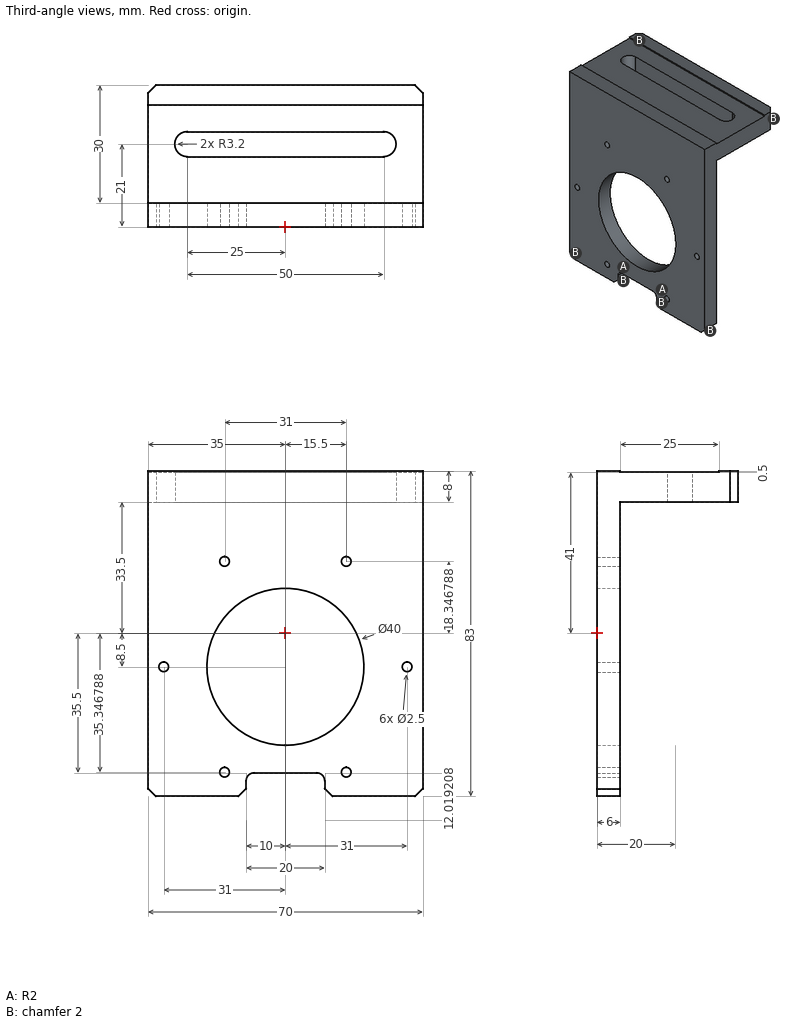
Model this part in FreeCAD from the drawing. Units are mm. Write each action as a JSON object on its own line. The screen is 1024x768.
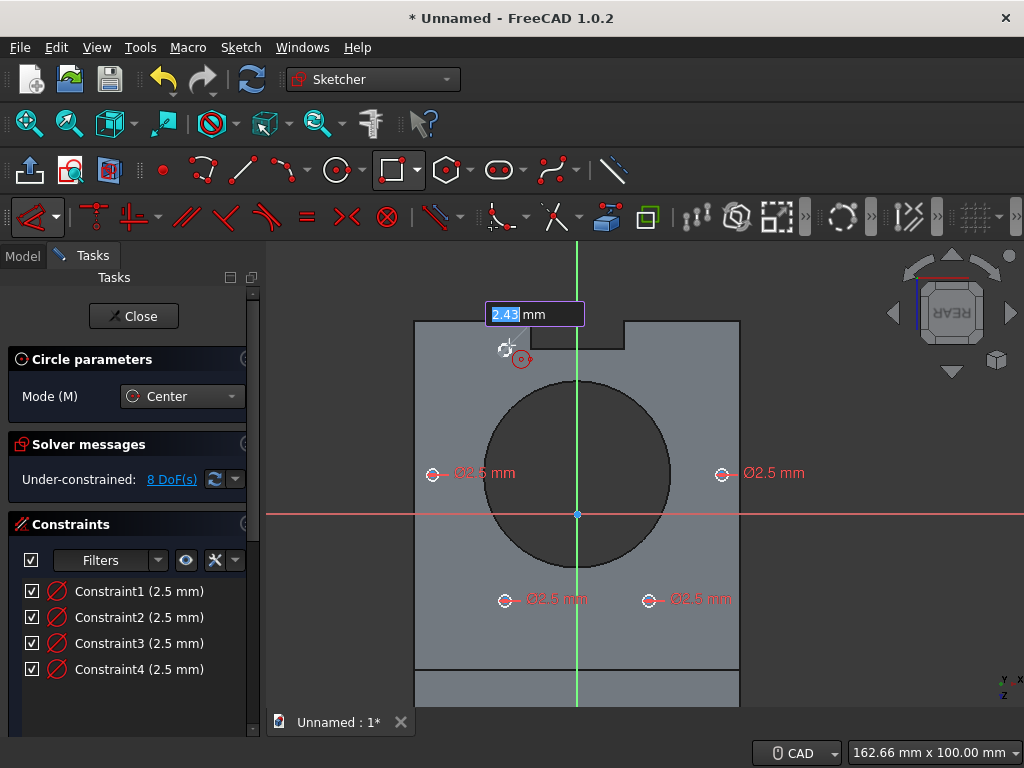
{"action": "type", "text": "2.5"}
{"action": "key", "text": "Return"}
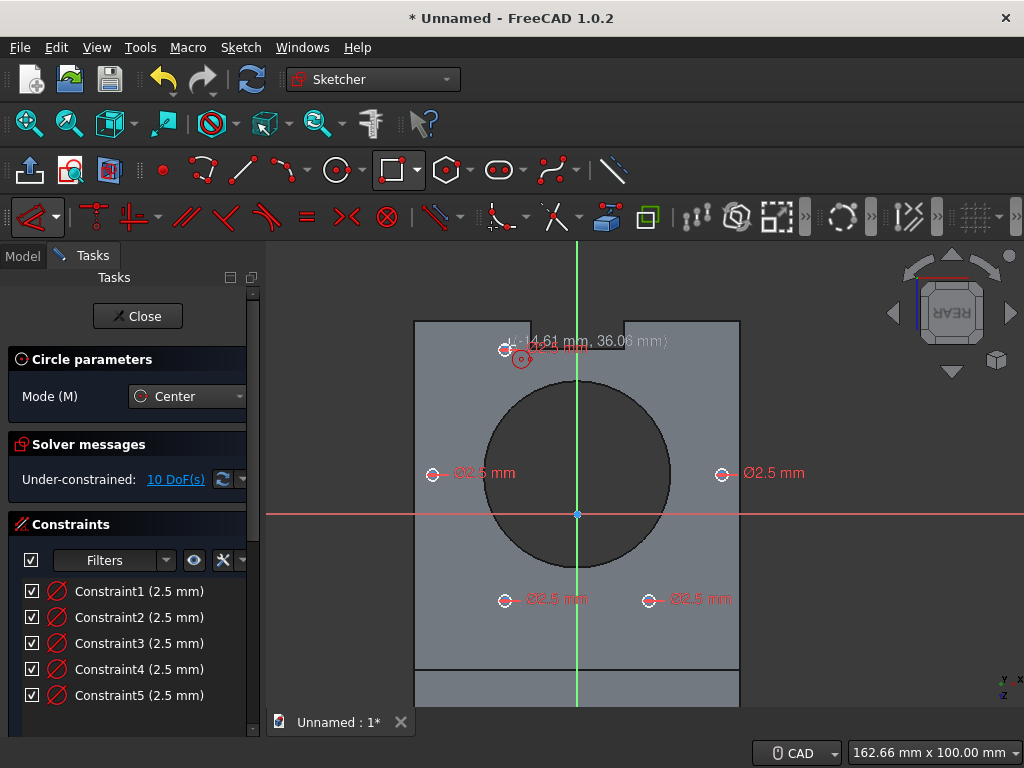
{"action": "scroll", "coordinate": [649, 349], "scroll_direction": "up", "scroll_amount": 7}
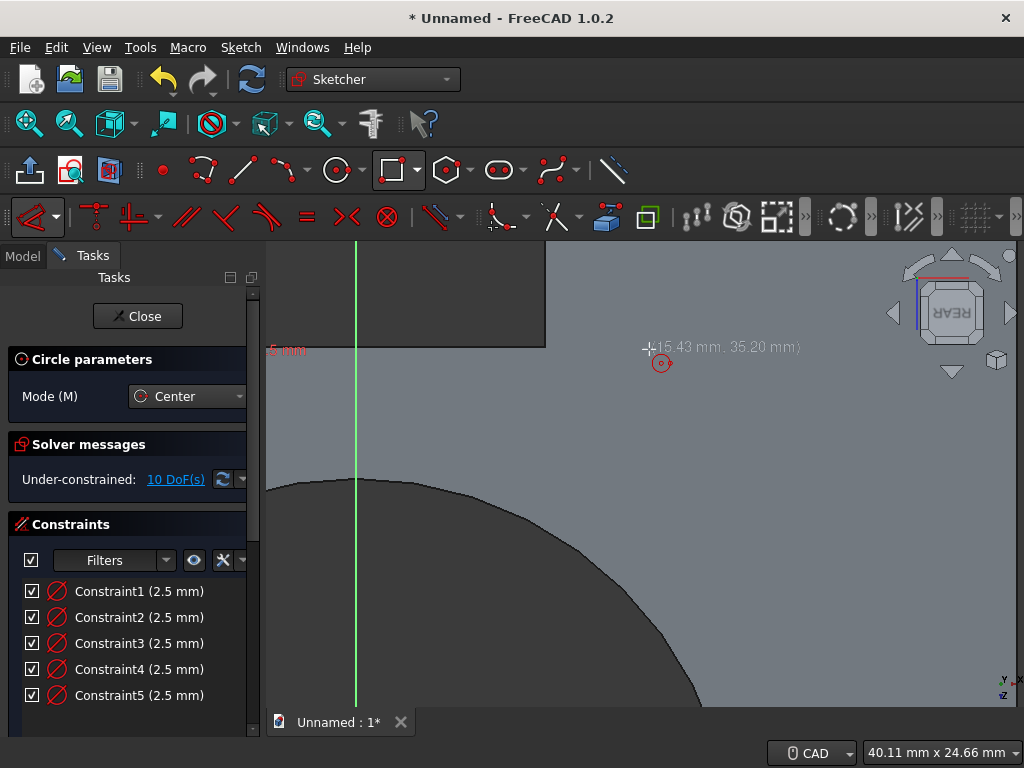
{"action": "scroll", "coordinate": [649, 349], "scroll_direction": "down", "scroll_amount": 7}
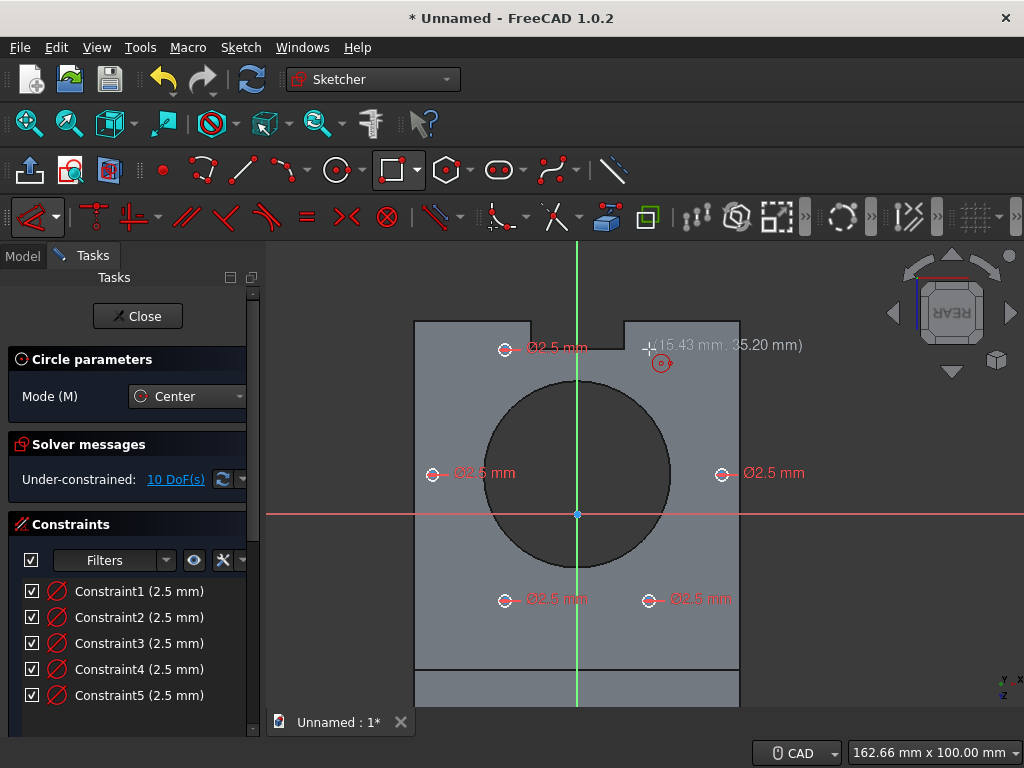
{"action": "left_click", "coordinate": [649, 349]}
{"action": "mouse_move", "coordinate": [653, 345]}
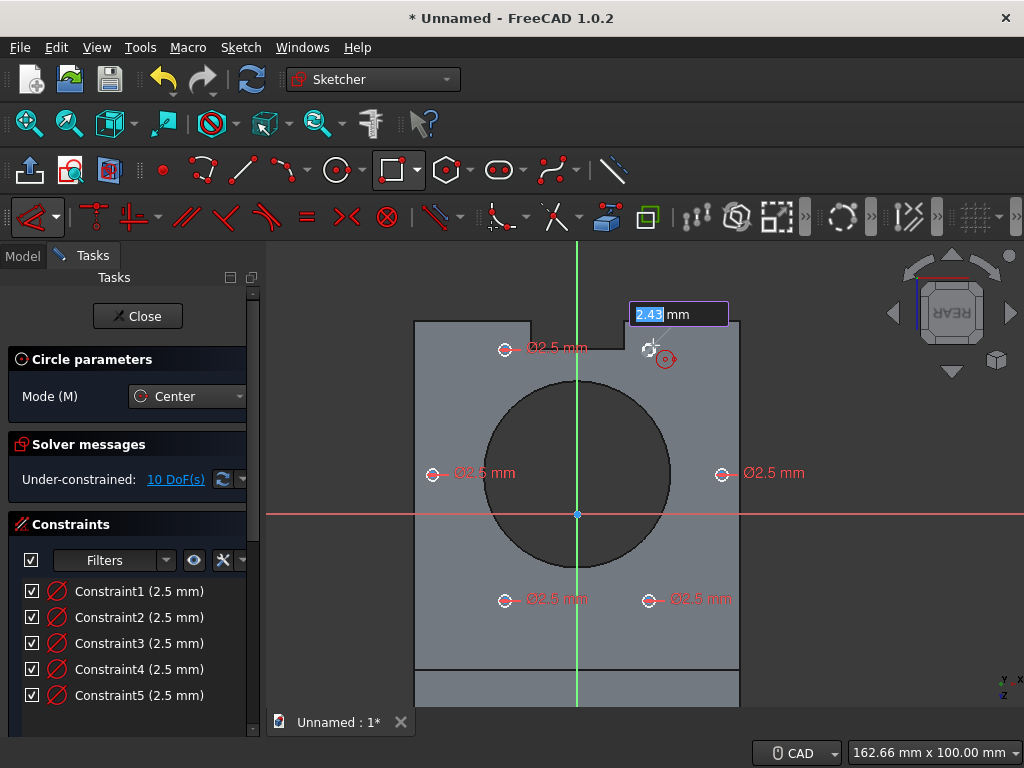
{"action": "type", "text": "2.5"}
{"action": "key", "text": "Return"}
{"action": "key", "text": "Escape"}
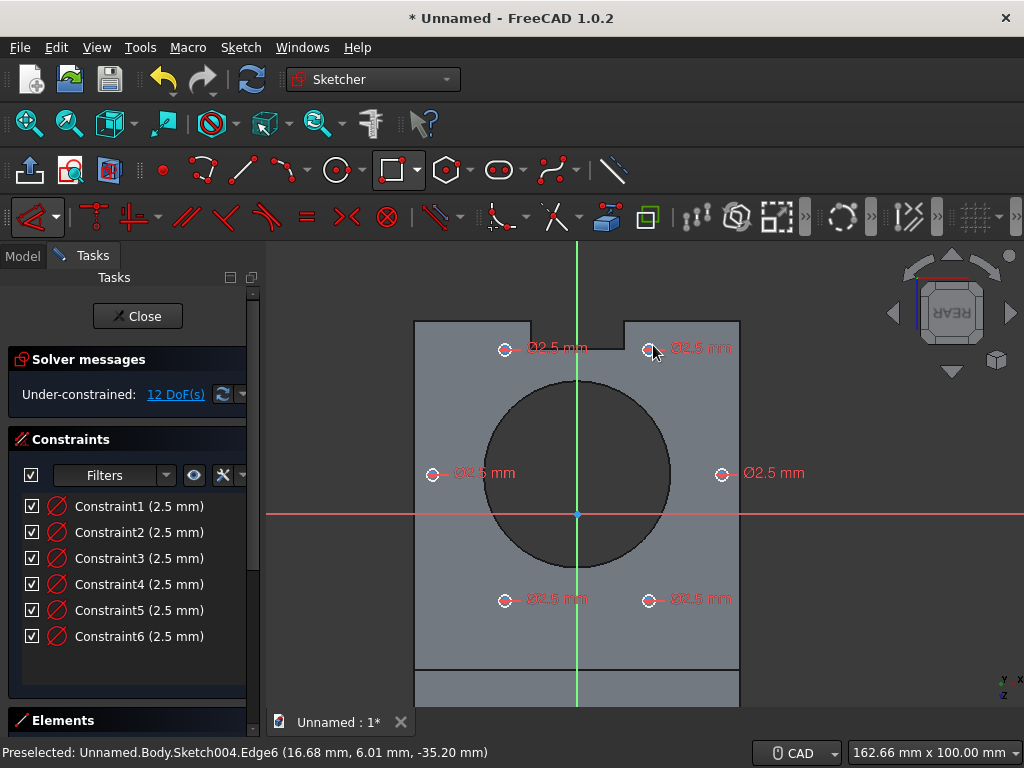
{"action": "left_click", "coordinate": [649, 601]}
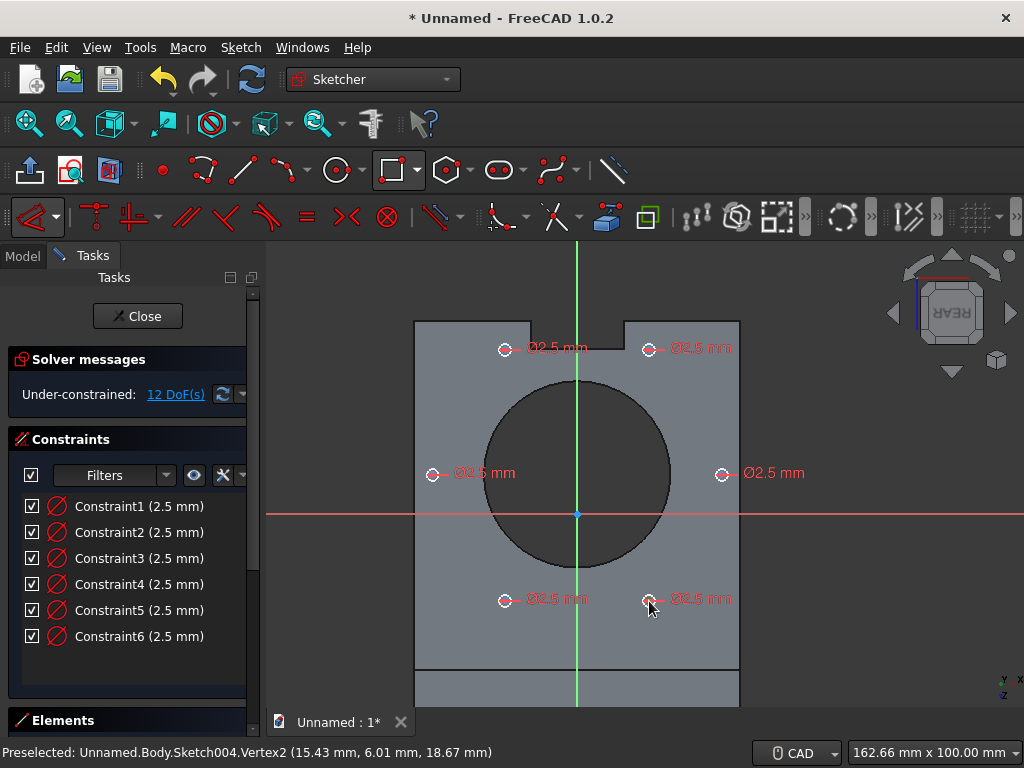
{"action": "left_click", "coordinate": [505, 601]}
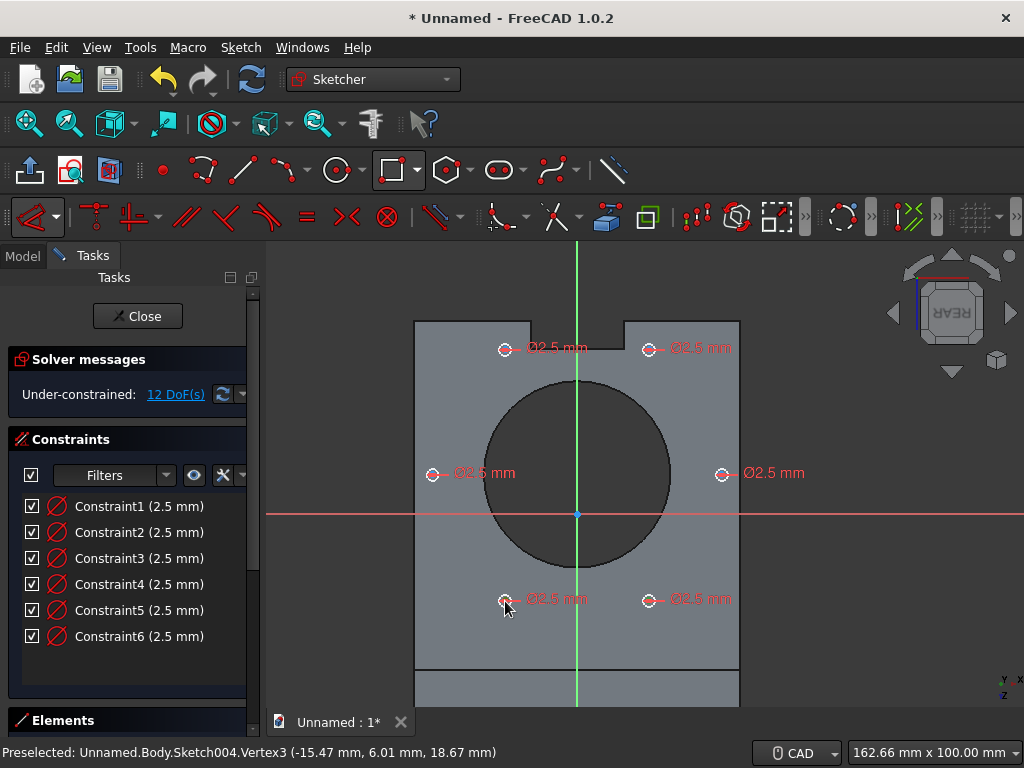
{"action": "left_click", "coordinate": [160, 218]}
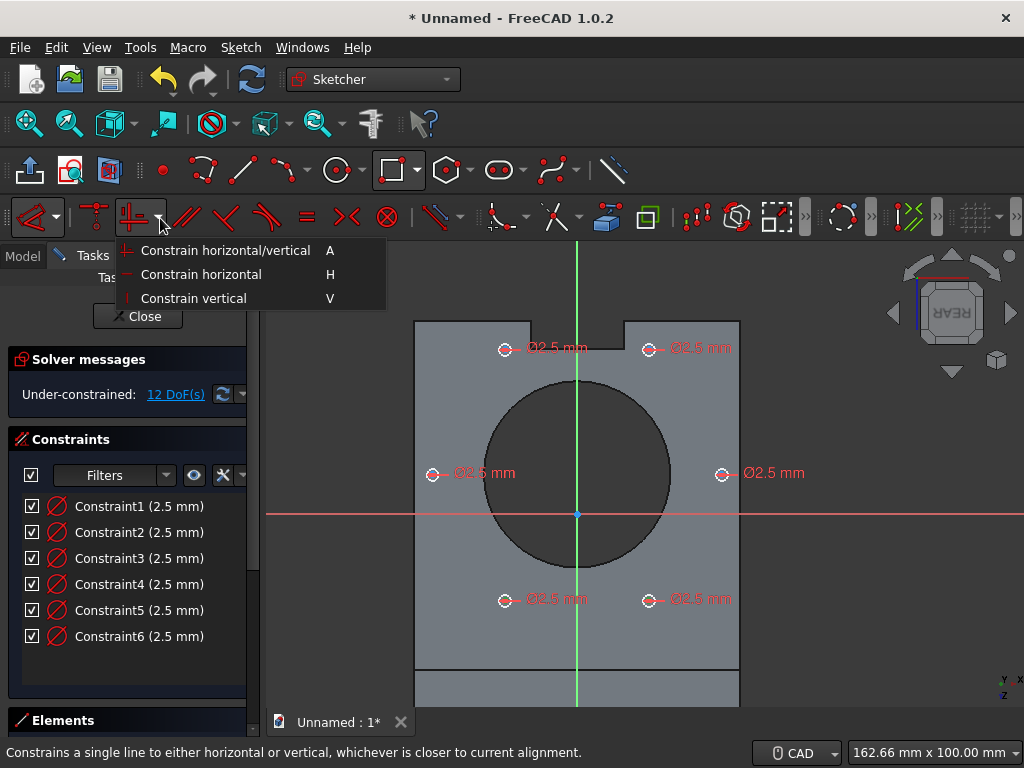
{"action": "left_click", "coordinate": [251, 274]}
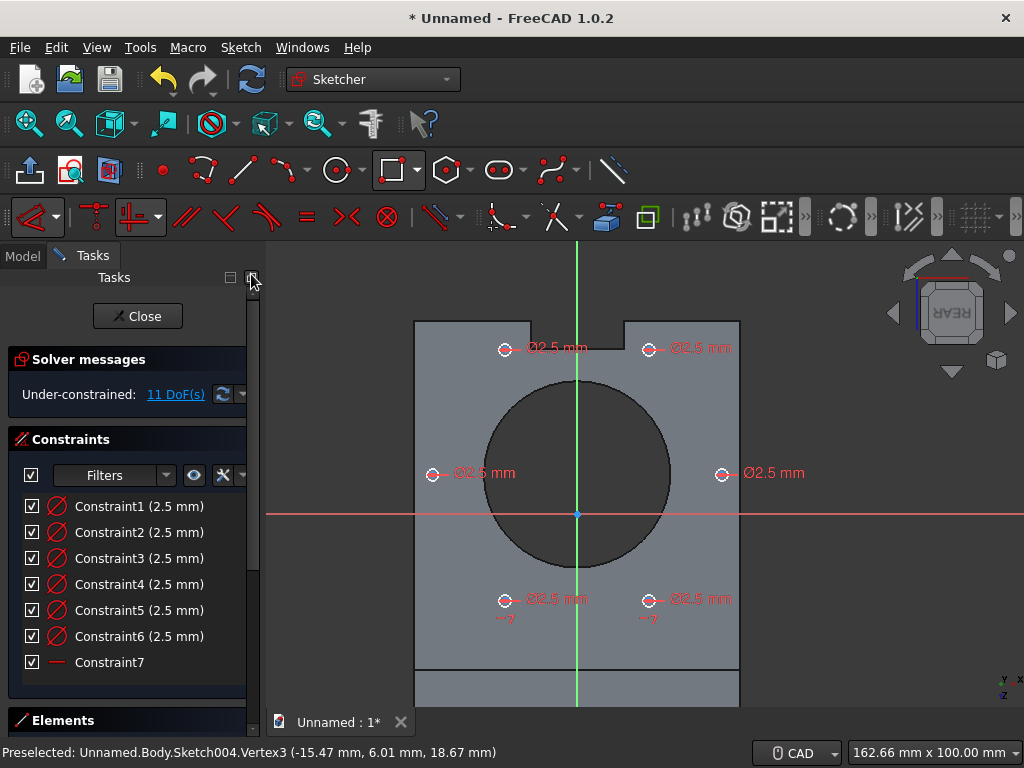
{"action": "left_click", "coordinate": [722, 475]}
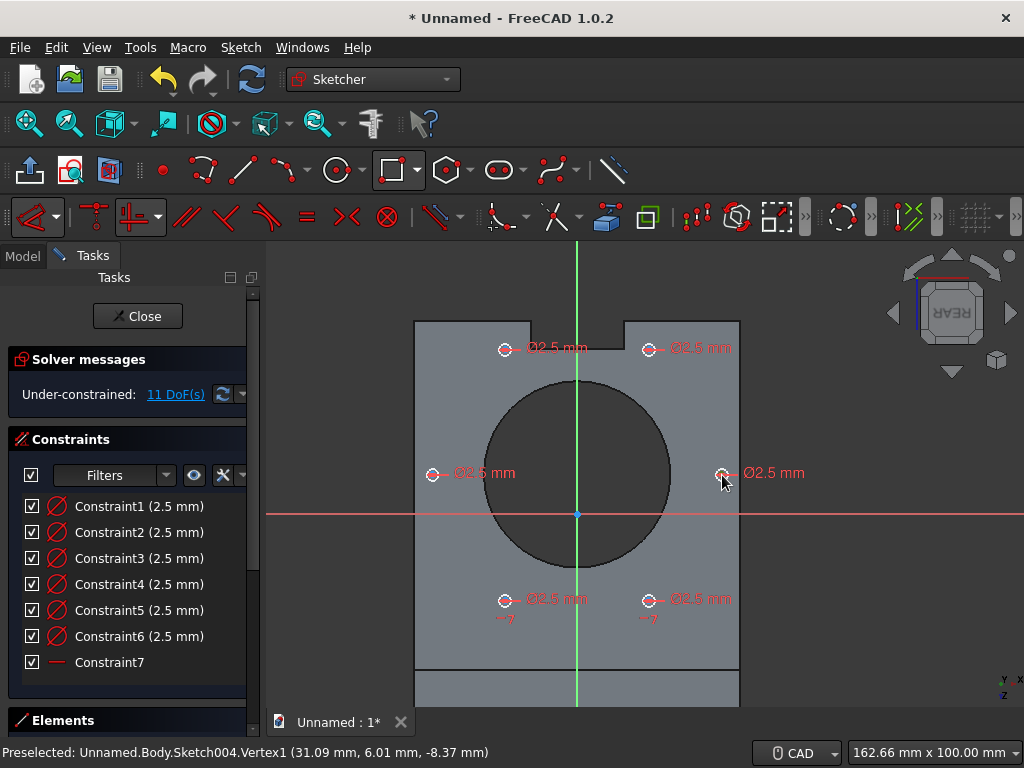
{"action": "left_click", "coordinate": [433, 475]}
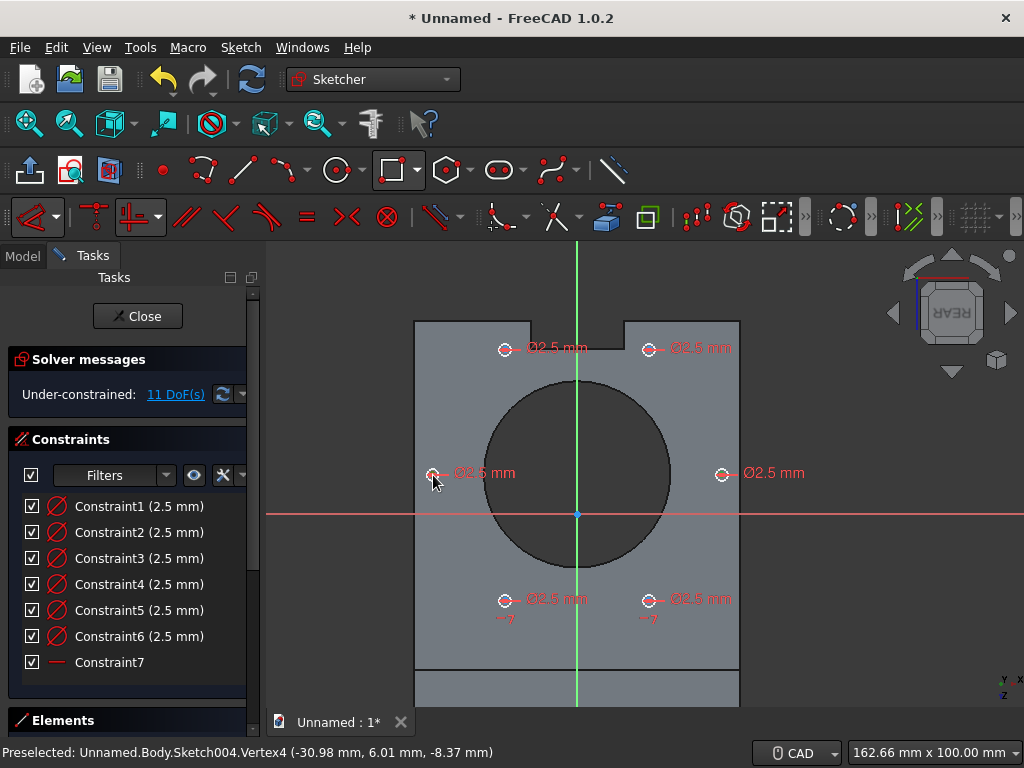
{"action": "key", "text": "h"}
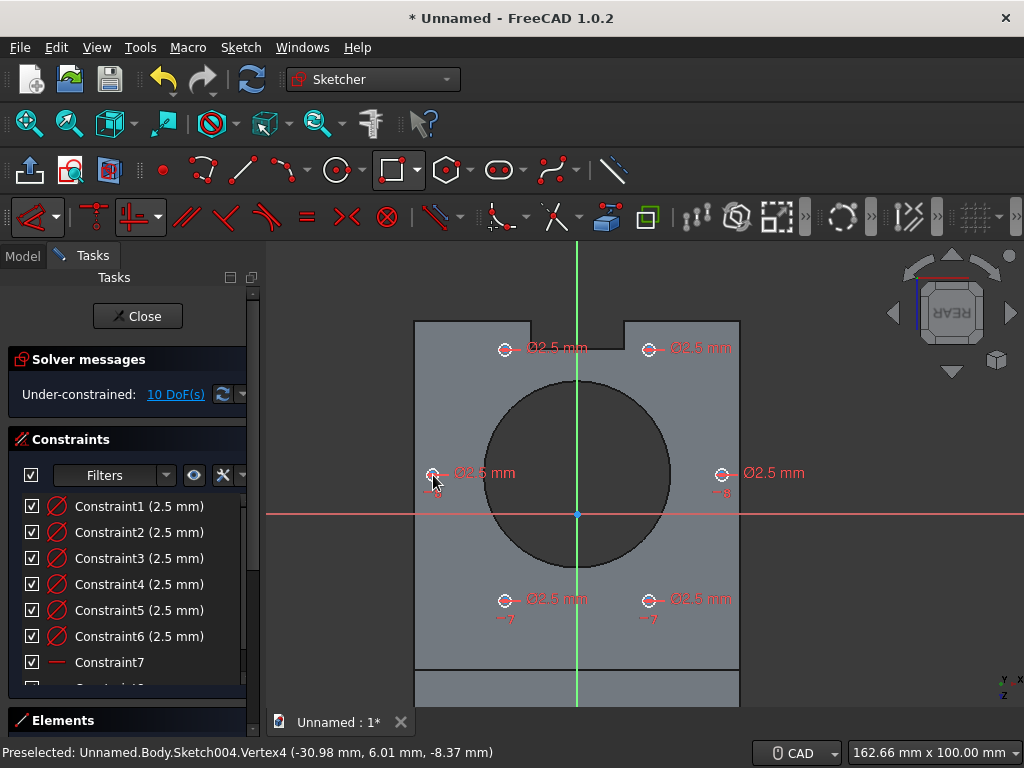
{"action": "left_click", "coordinate": [505, 601]}